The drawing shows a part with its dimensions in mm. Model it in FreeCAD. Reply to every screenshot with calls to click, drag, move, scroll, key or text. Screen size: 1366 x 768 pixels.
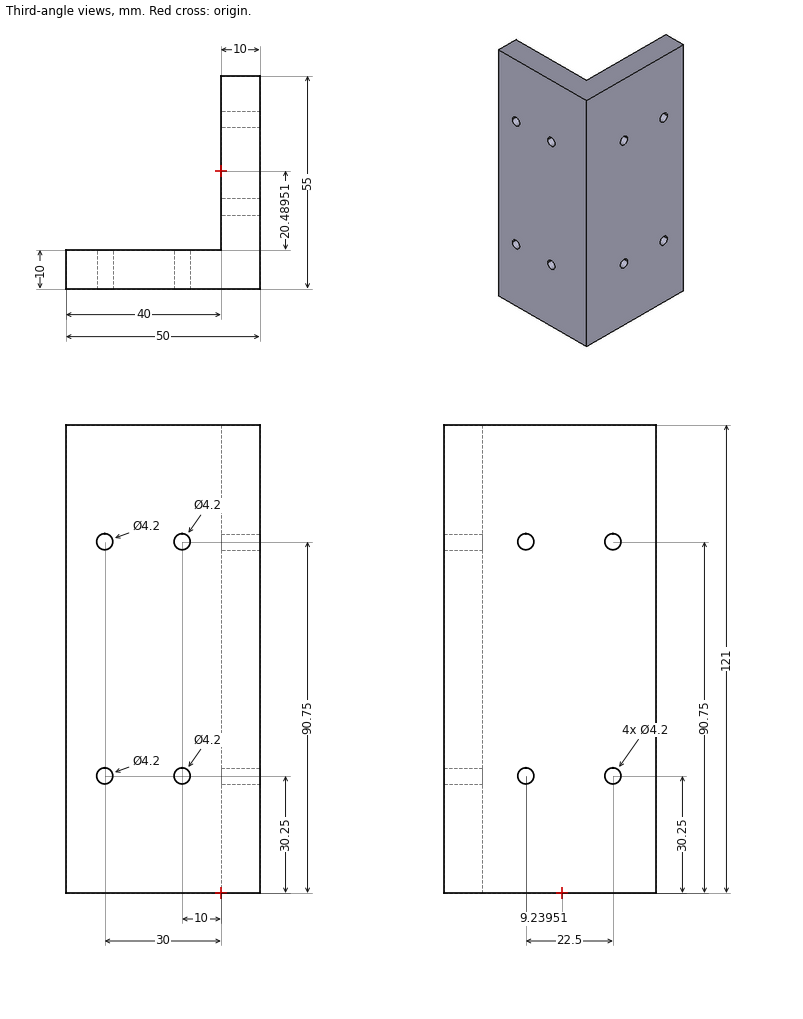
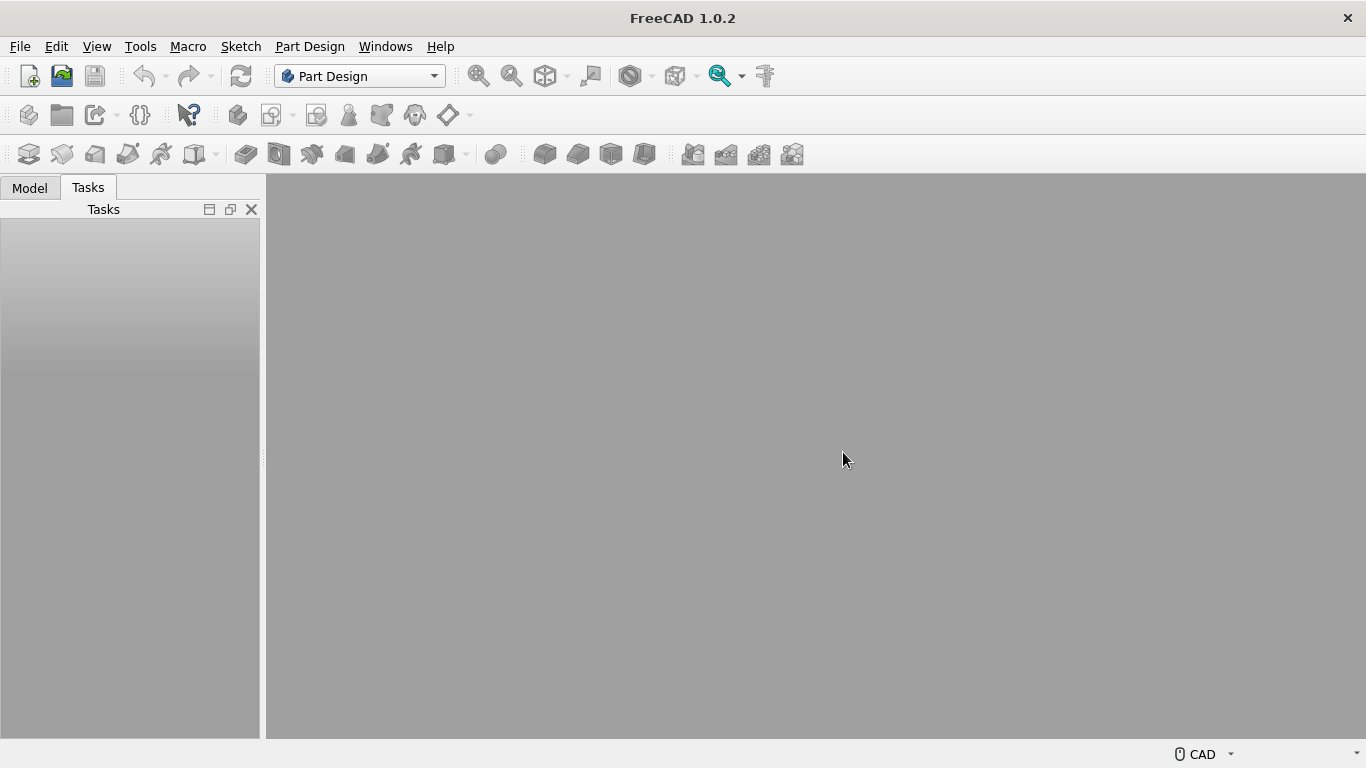
click(29, 76)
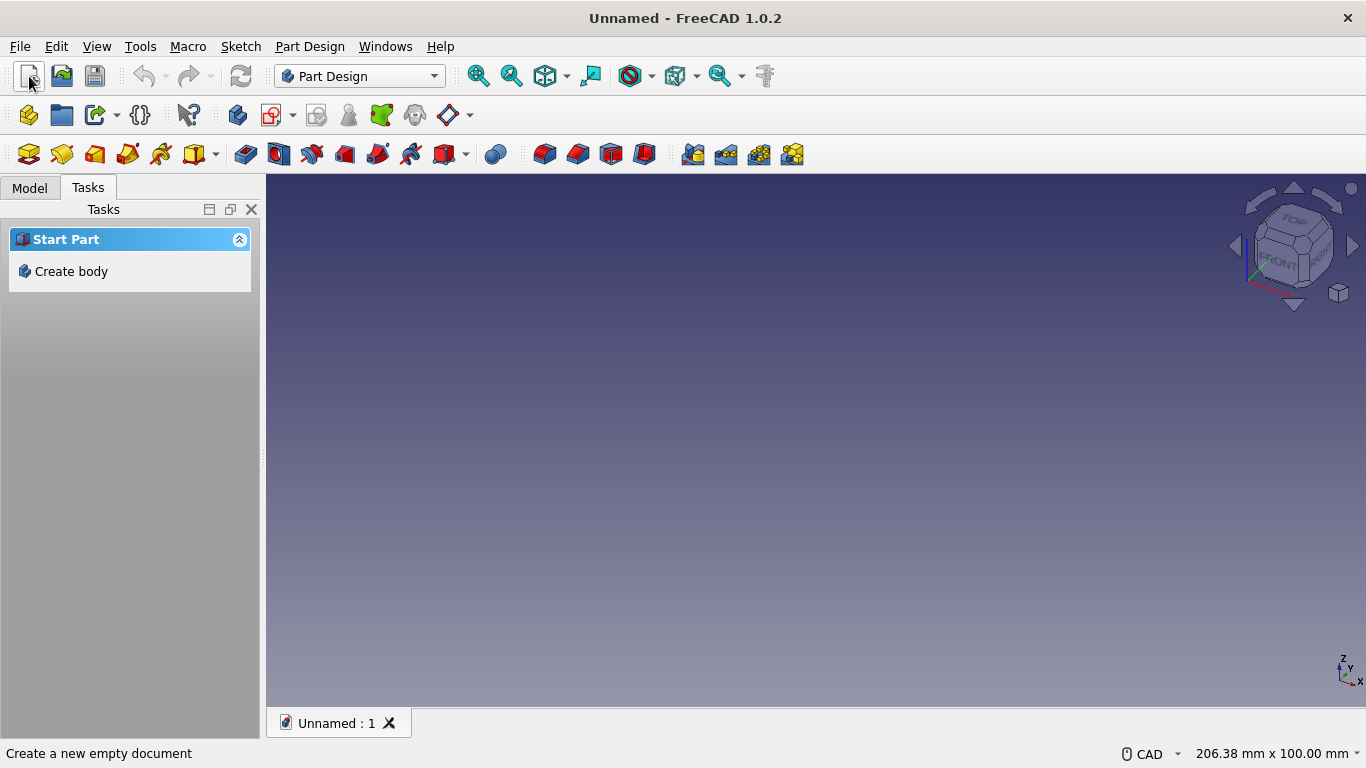
click(270, 116)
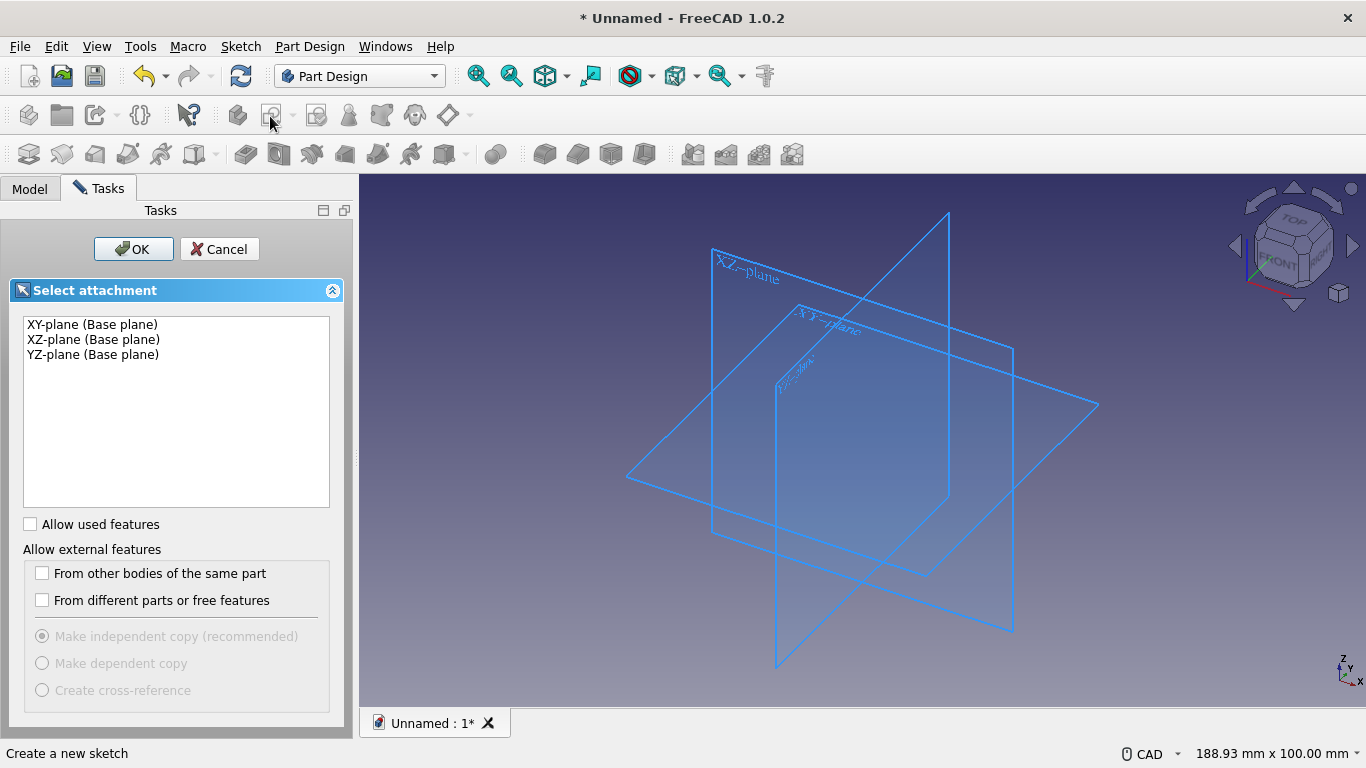
click(84, 324)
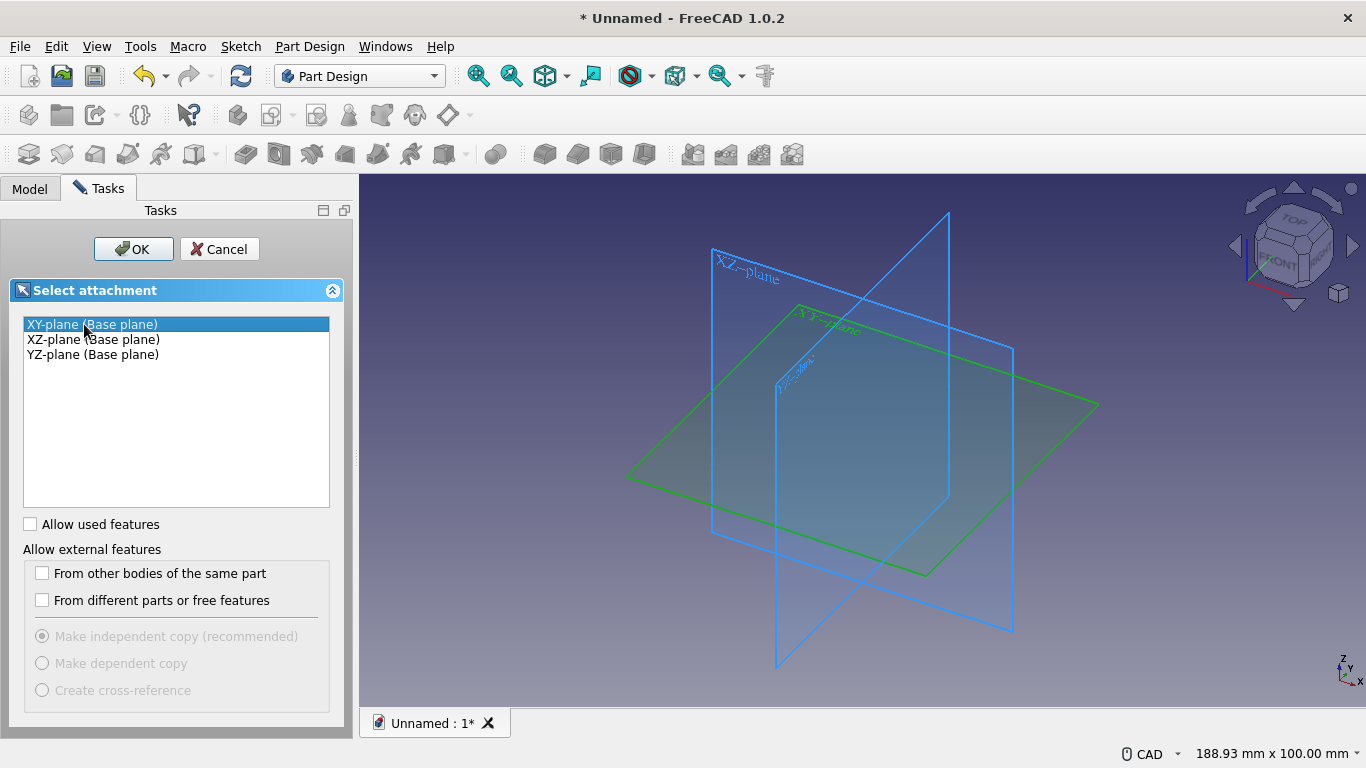
click(134, 249)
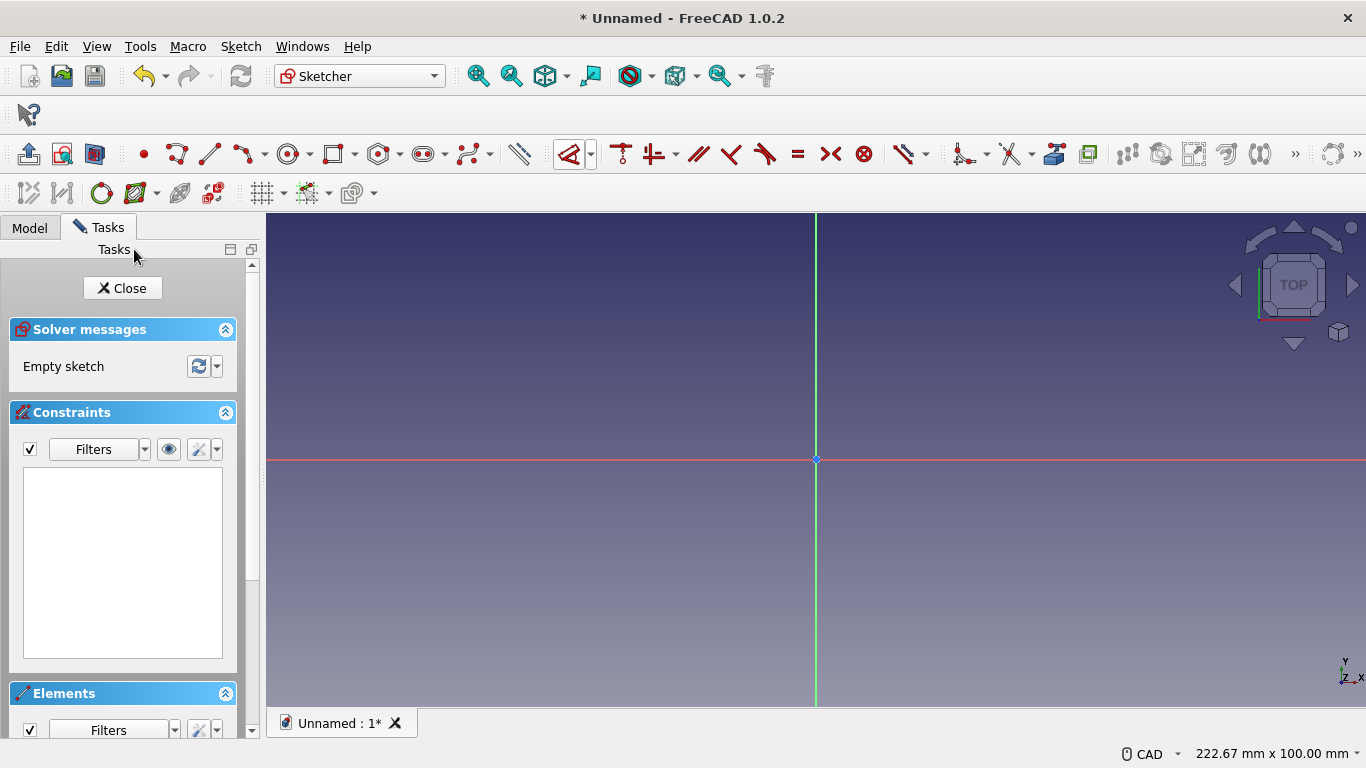
click(177, 154)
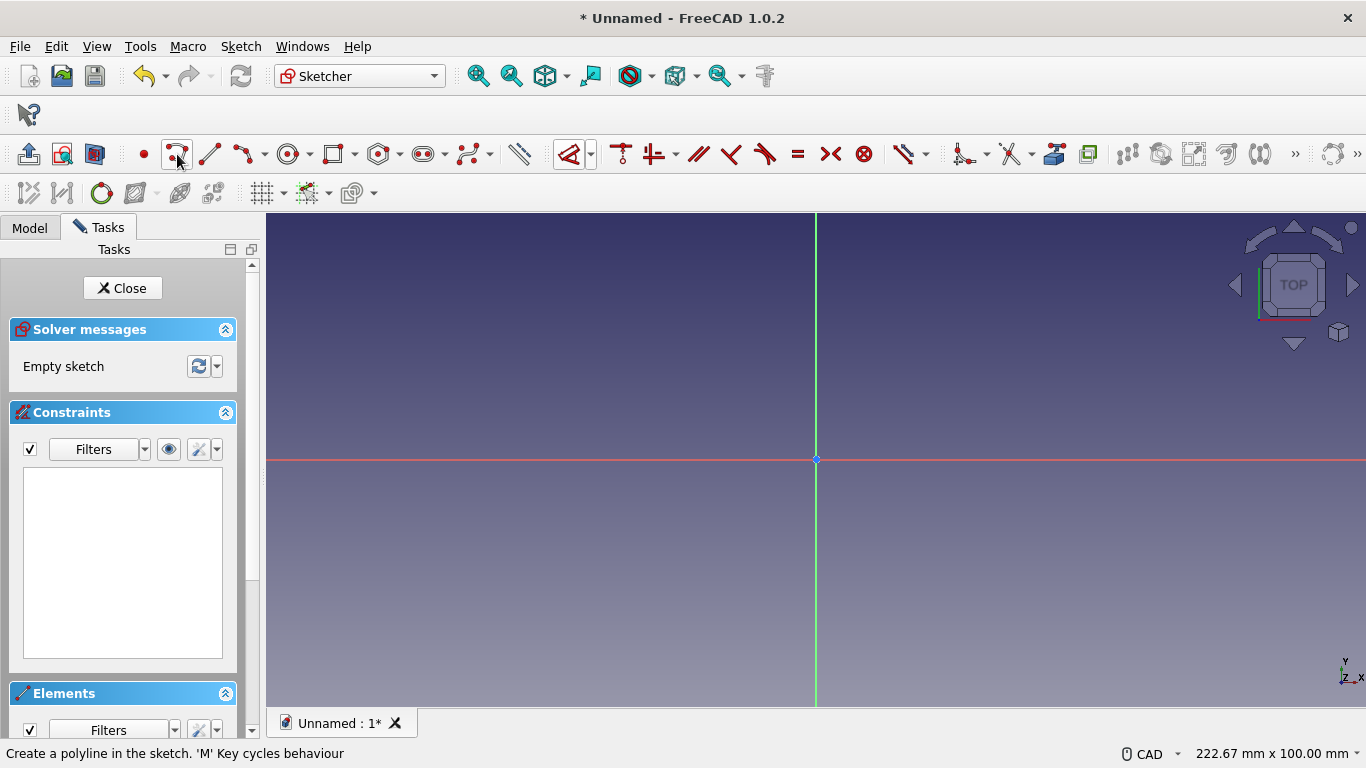
click(816, 561)
click(618, 561)
click(618, 611)
click(865, 611)
click(865, 339)
click(807, 339)
click(816, 562)
key(Escape)
key(Escape)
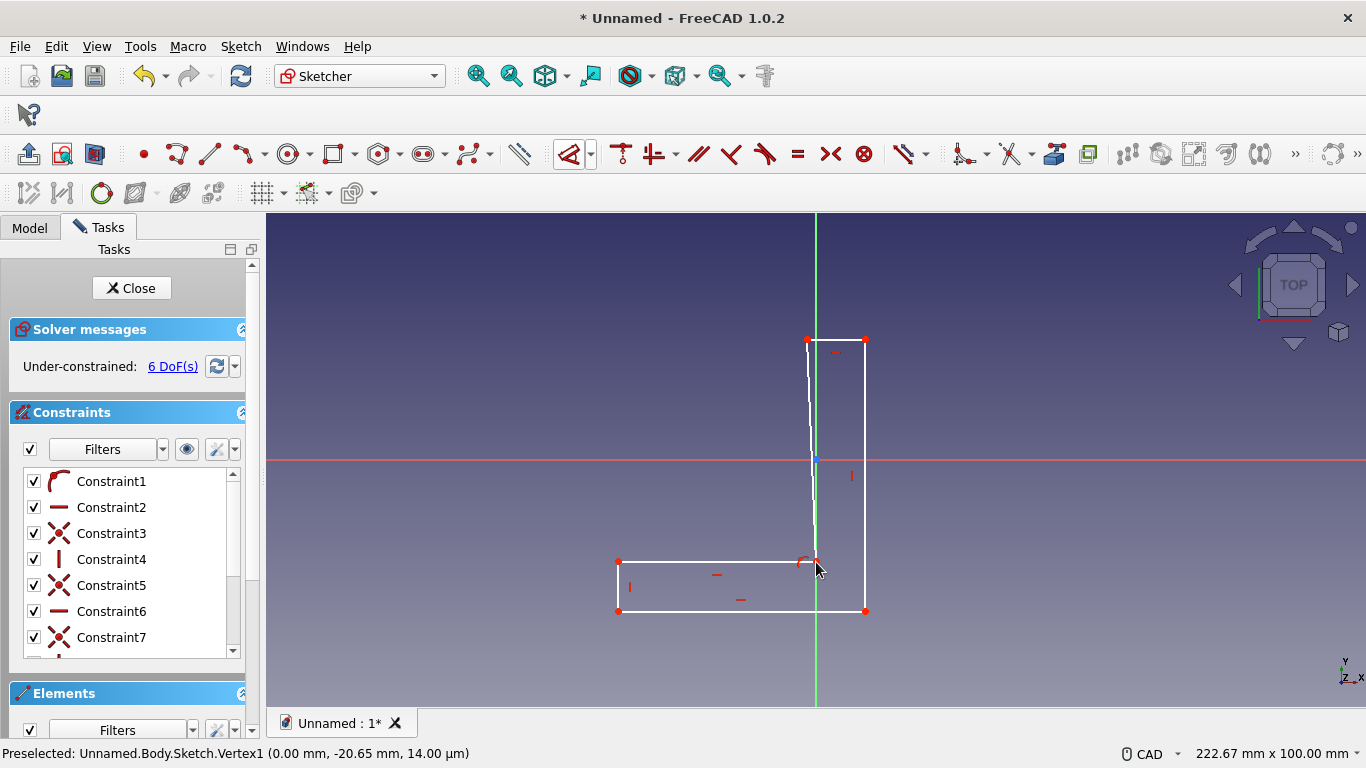
click(813, 495)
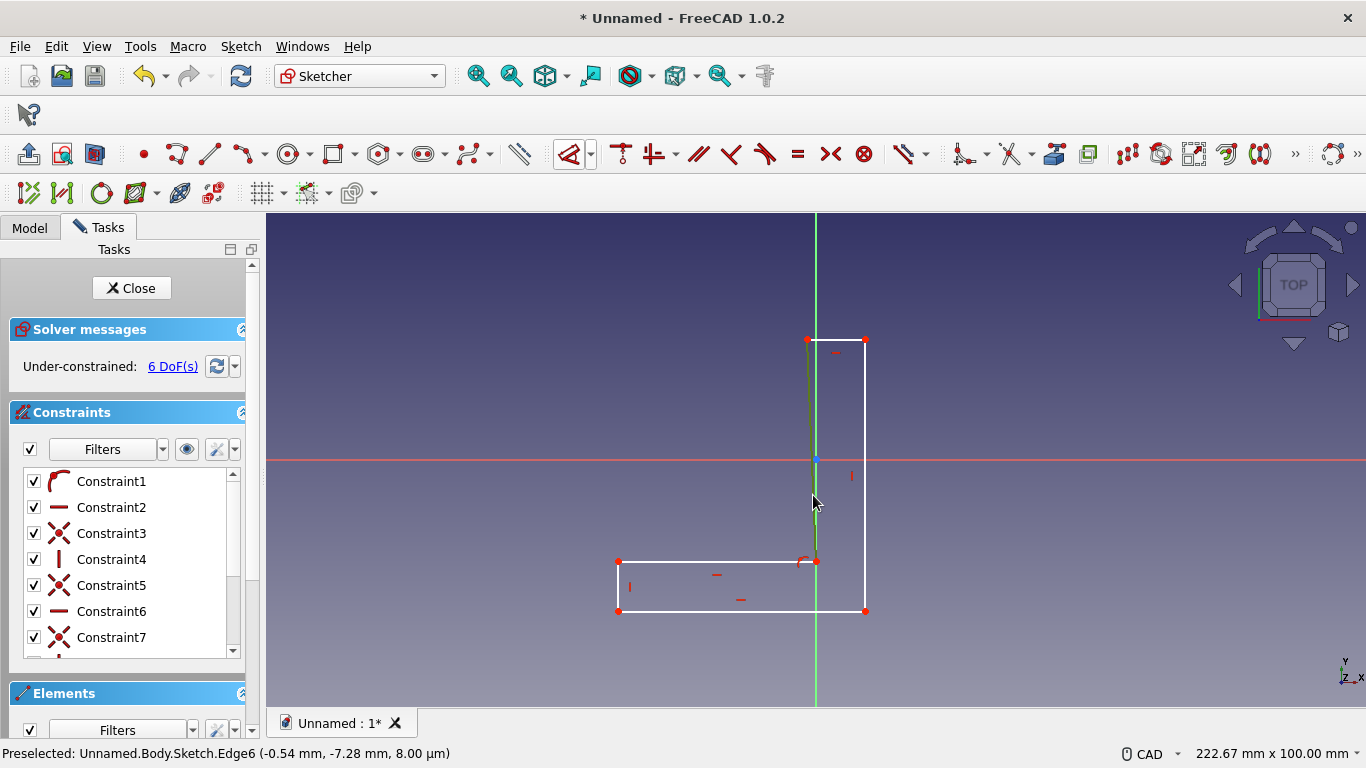
key(v)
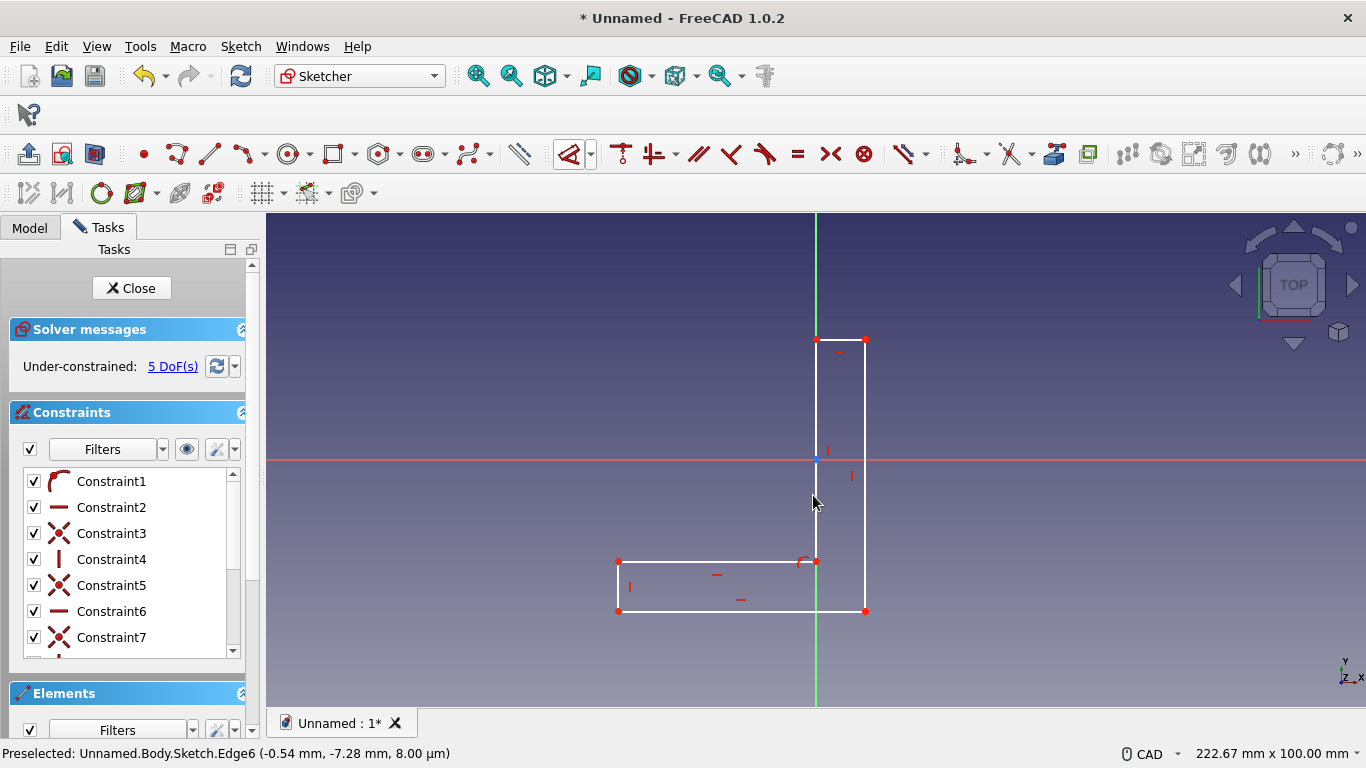
click(568, 154)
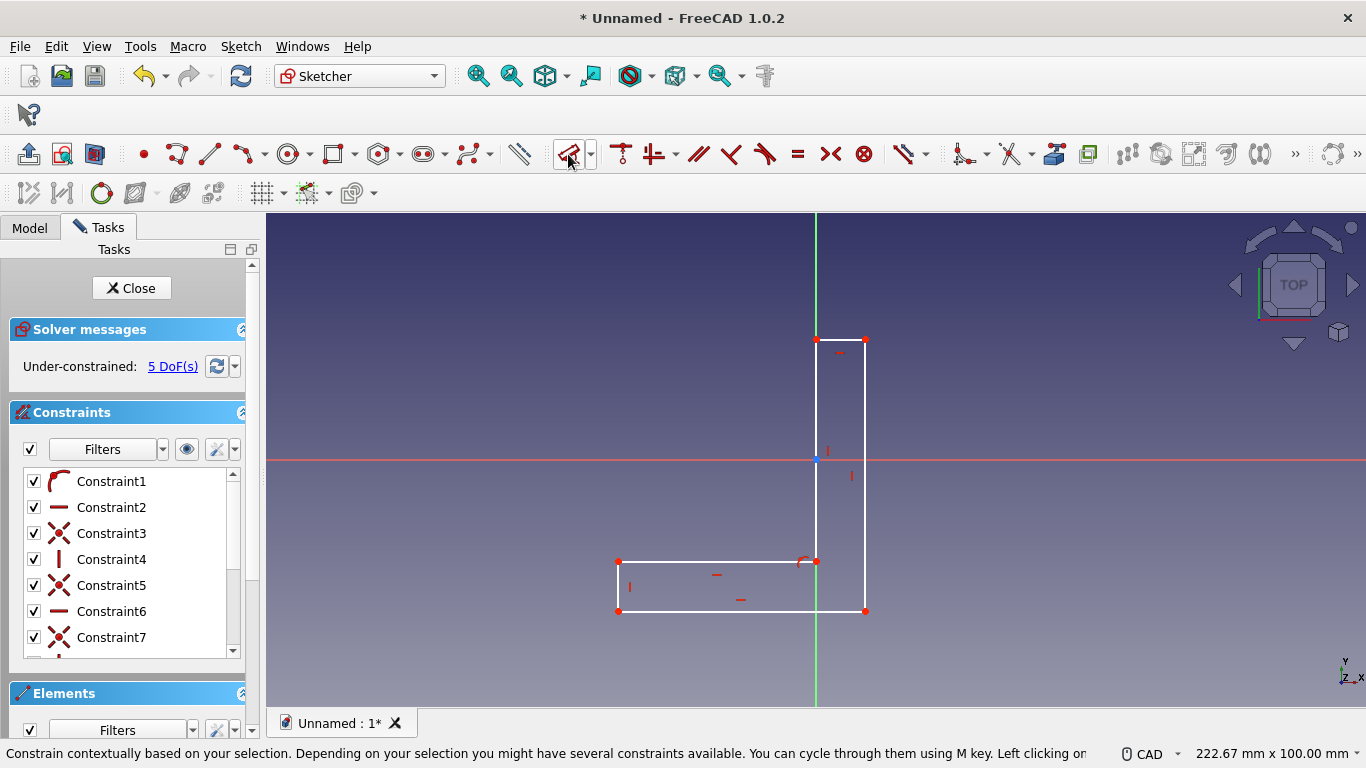
click(757, 562)
click(717, 596)